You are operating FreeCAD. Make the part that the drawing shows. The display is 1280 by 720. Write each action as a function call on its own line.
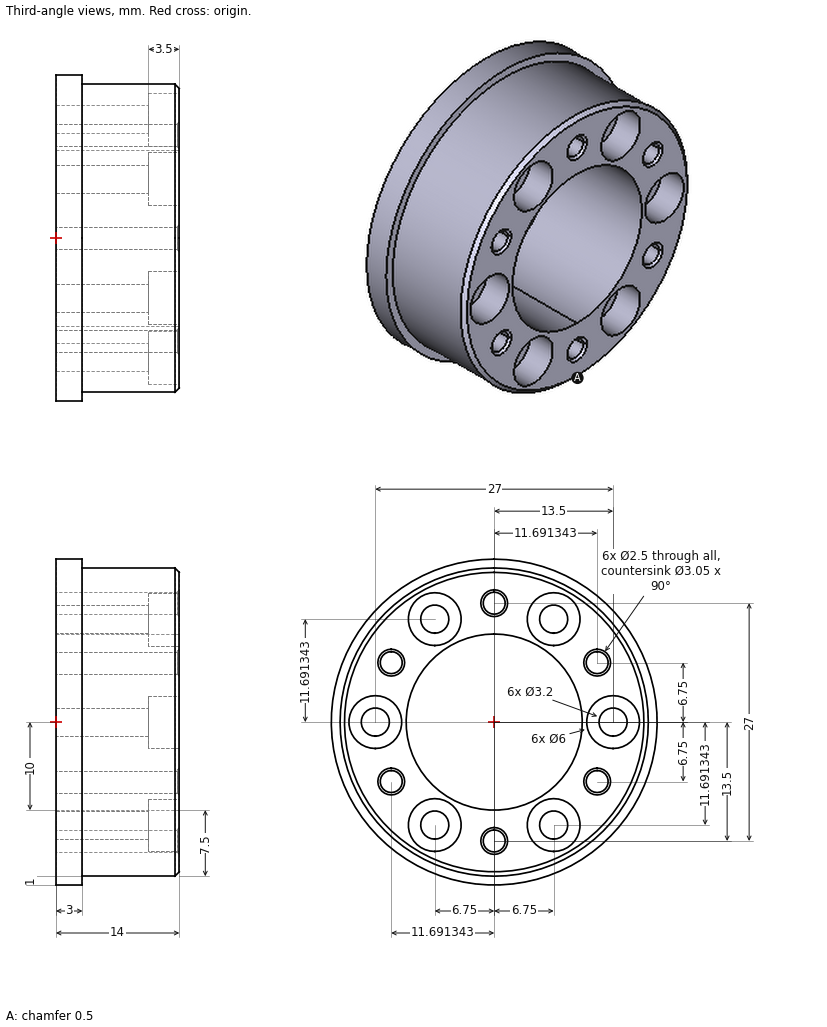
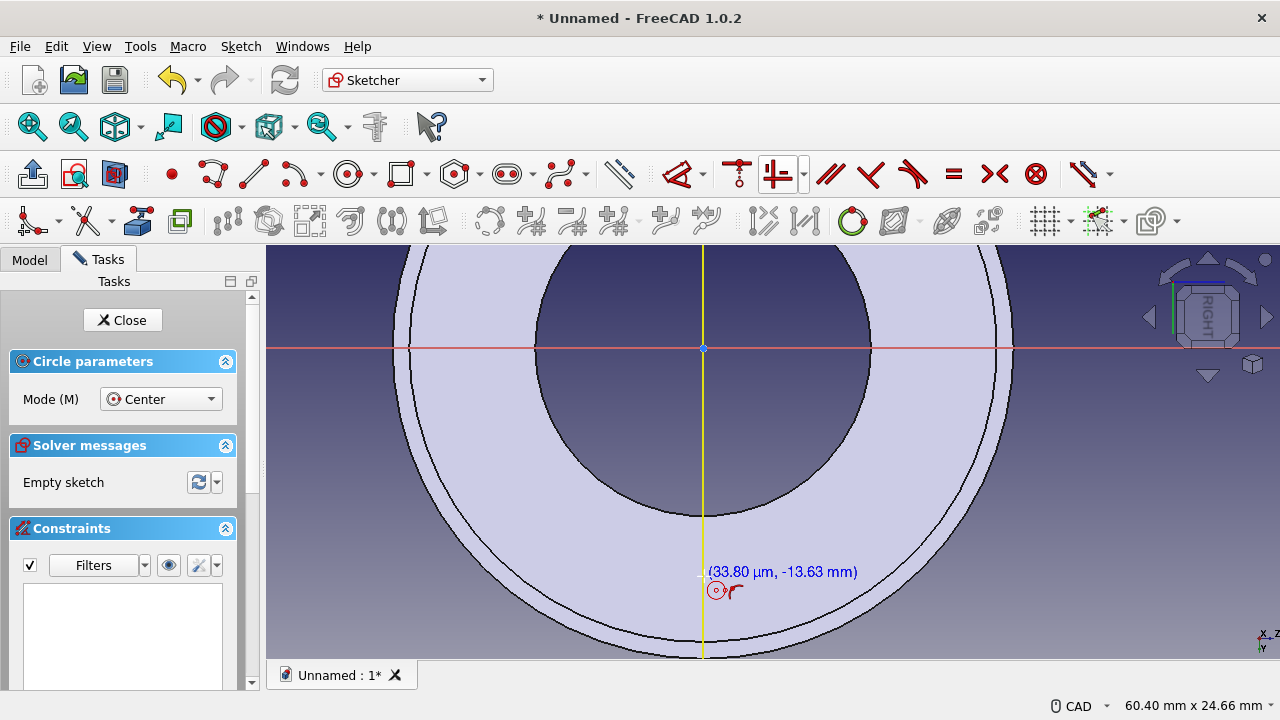
click(703, 575)
click(722, 556)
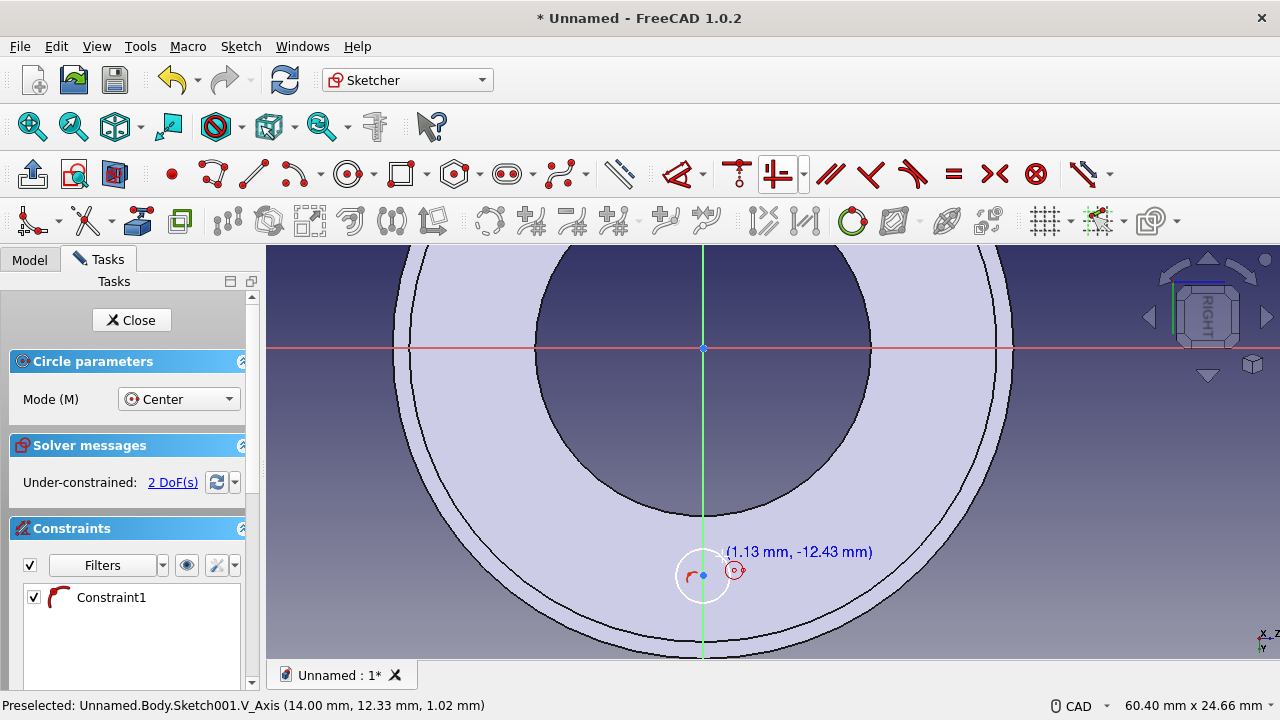
click(507, 462)
click(526, 443)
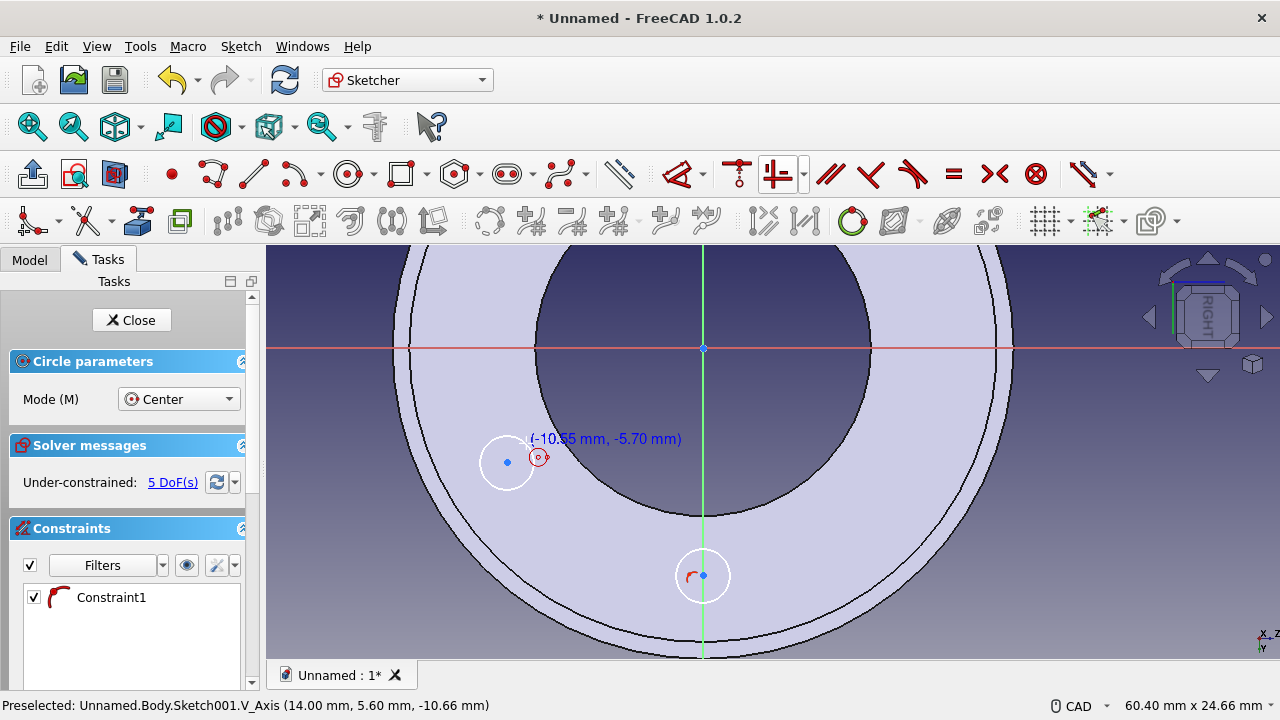
scroll(706, 578, down, 3)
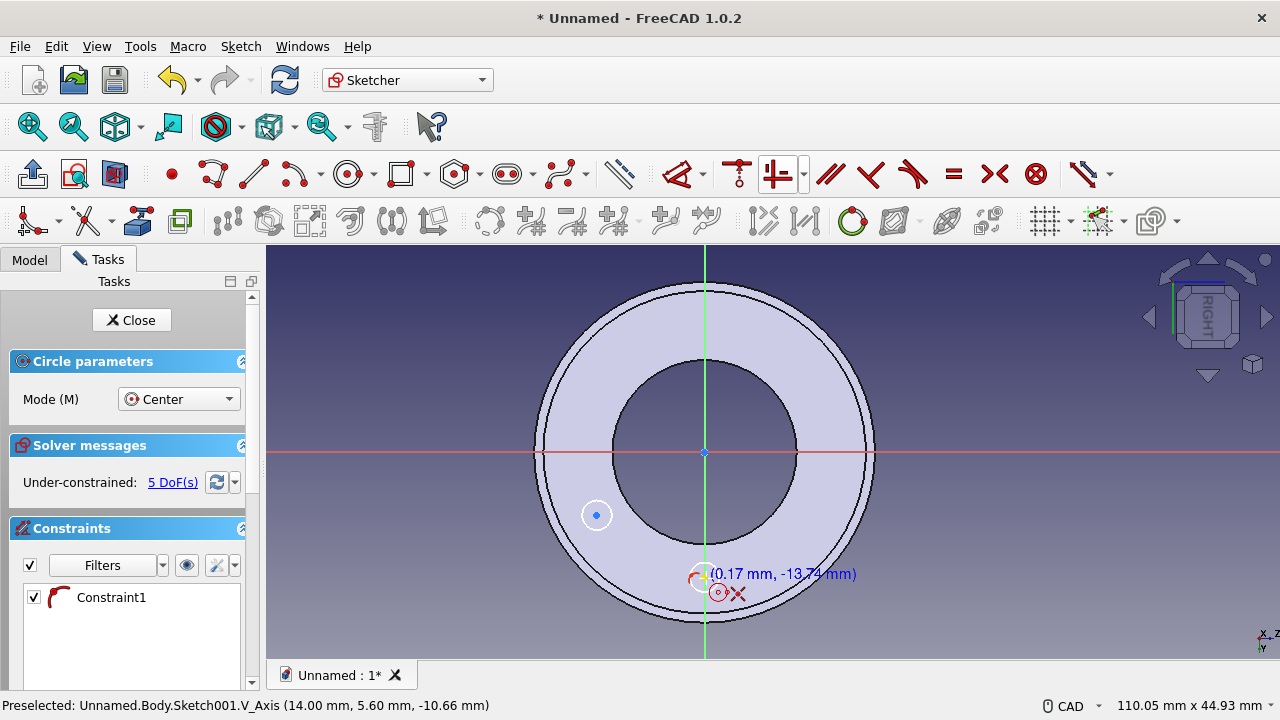
scroll(597, 390, up, 3)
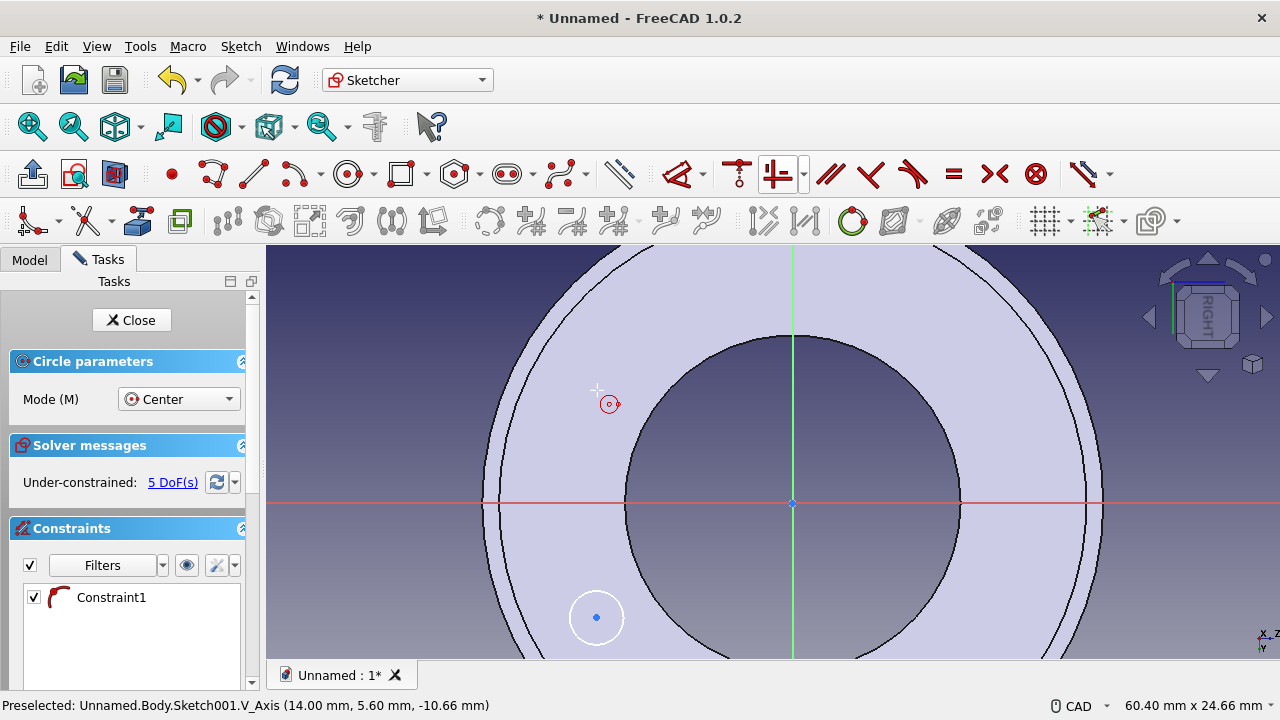
click(596, 390)
click(615, 371)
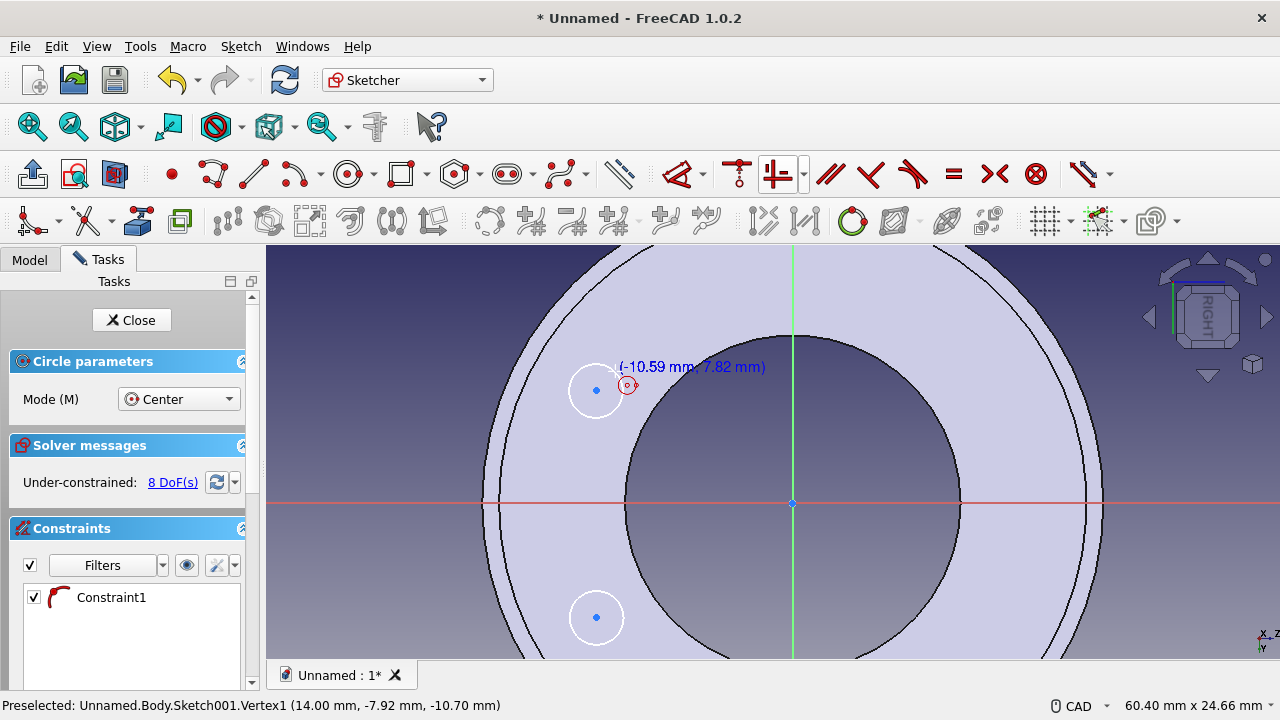
click(793, 277)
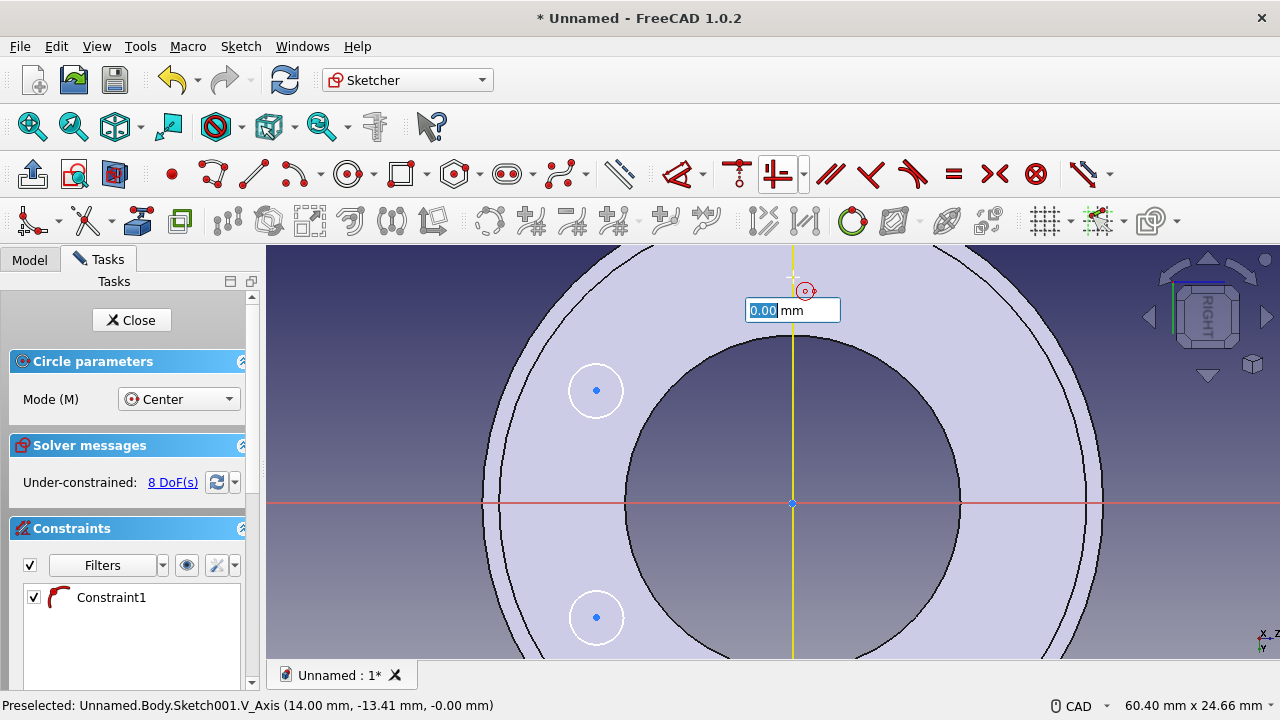
scroll(597, 390, down, 3)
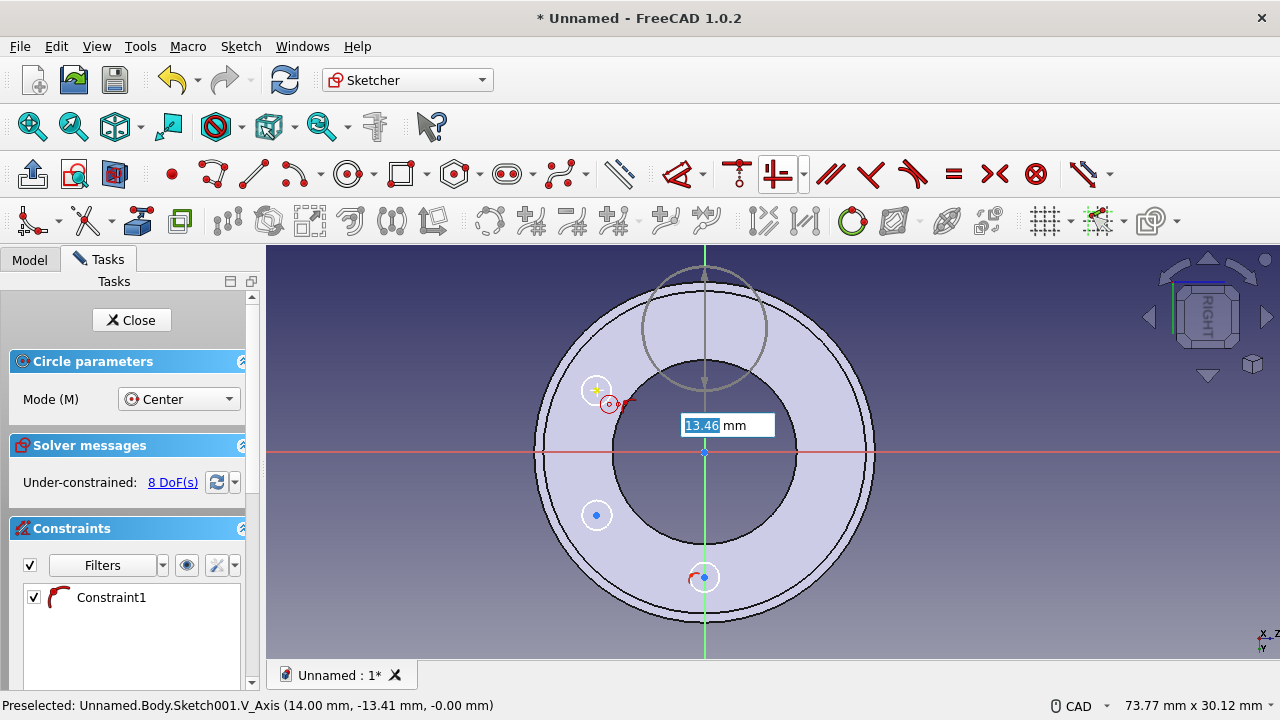
scroll(715, 317, up, 3)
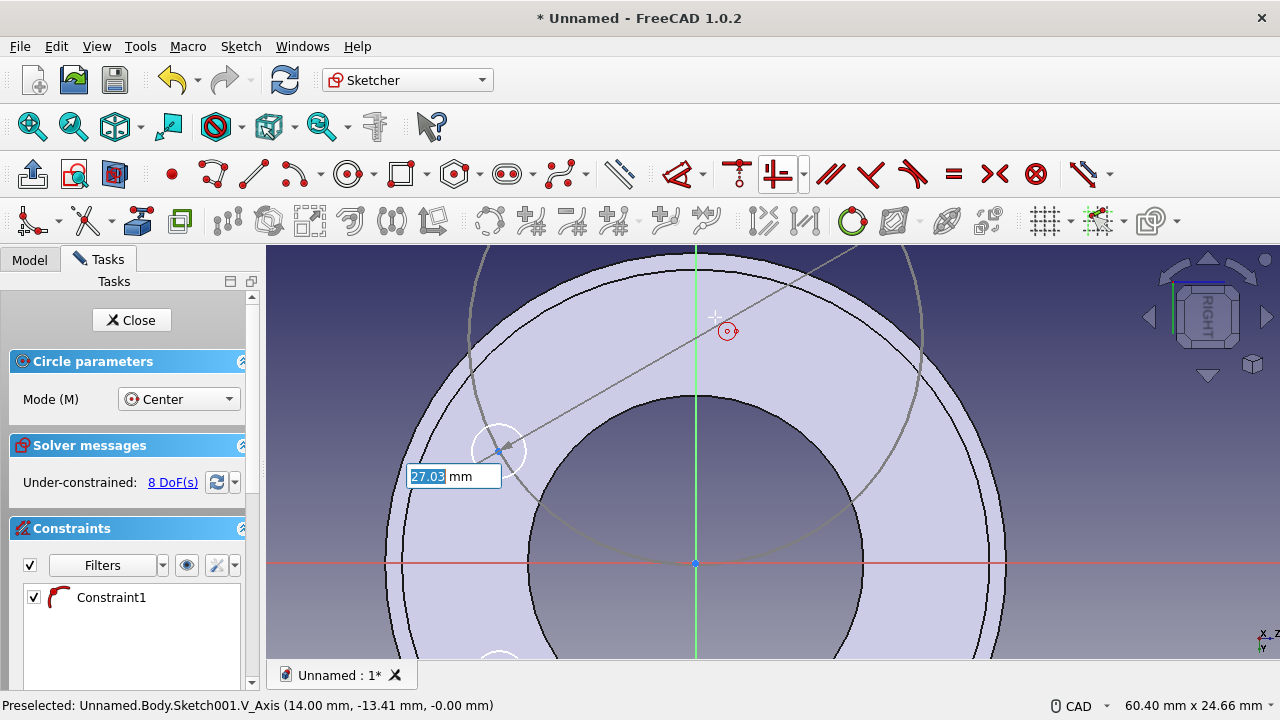
click(715, 318)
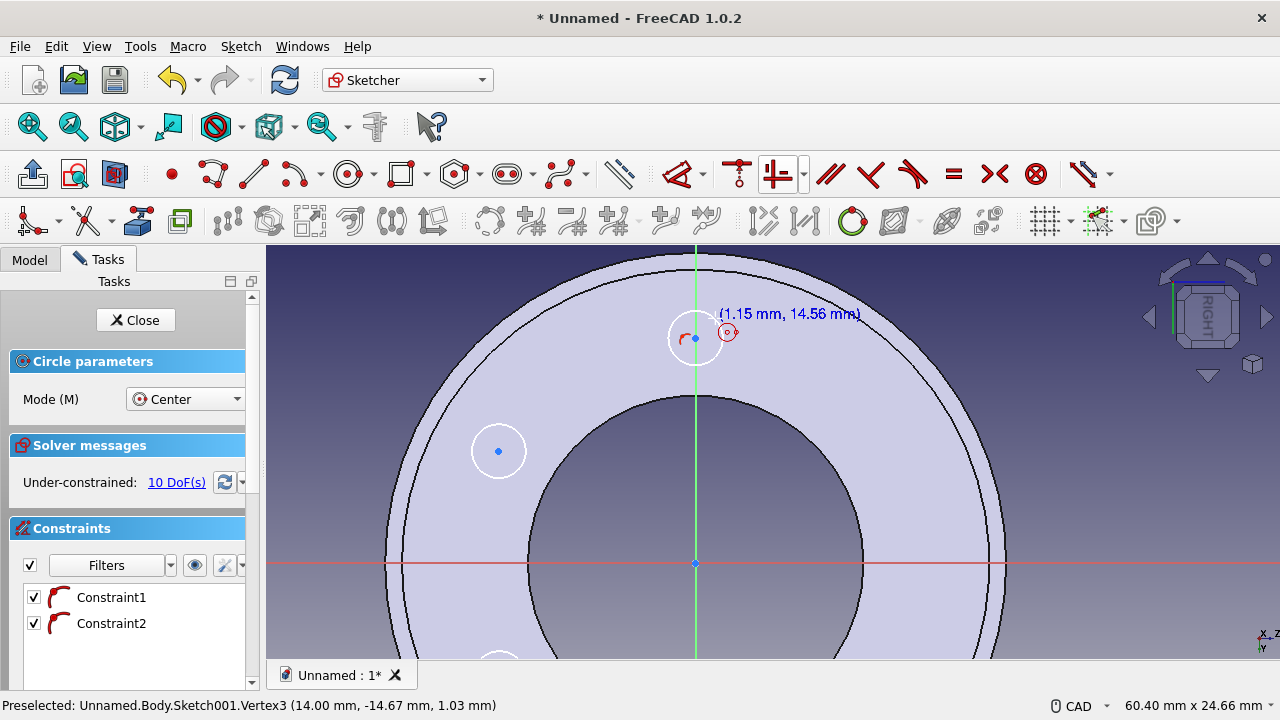
click(892, 450)
click(911, 431)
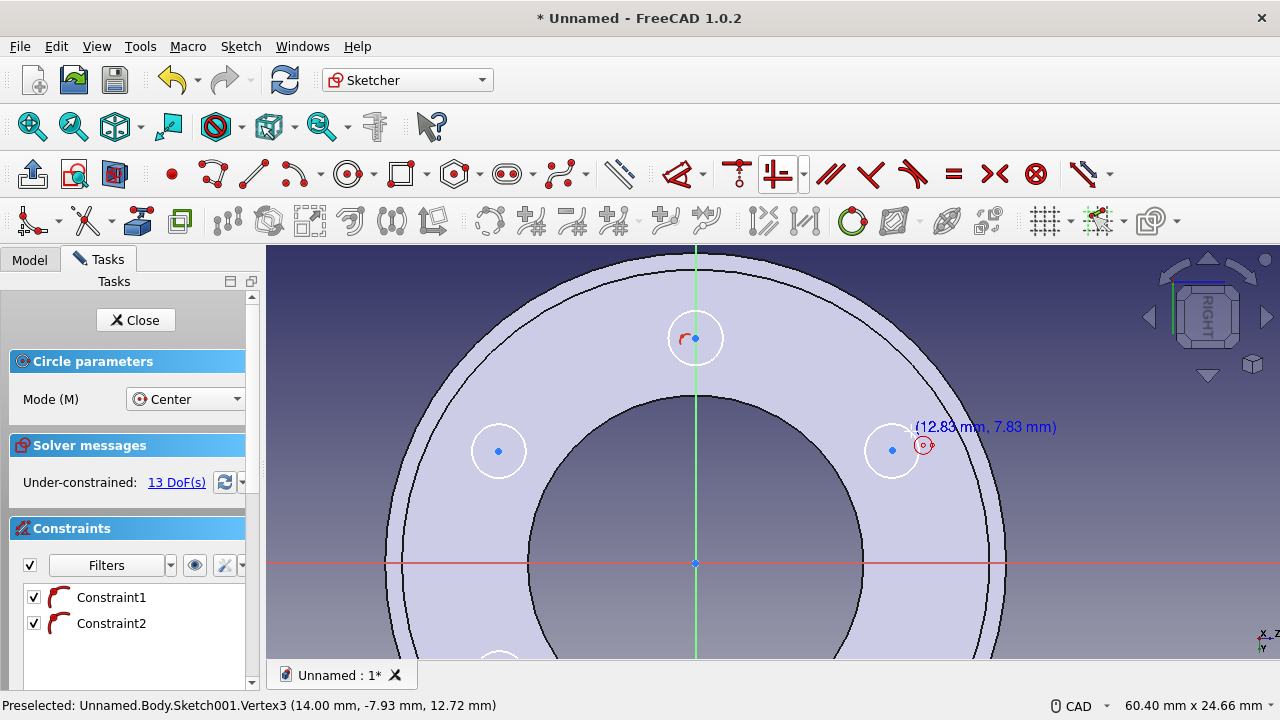
scroll(715, 317, down, 3)